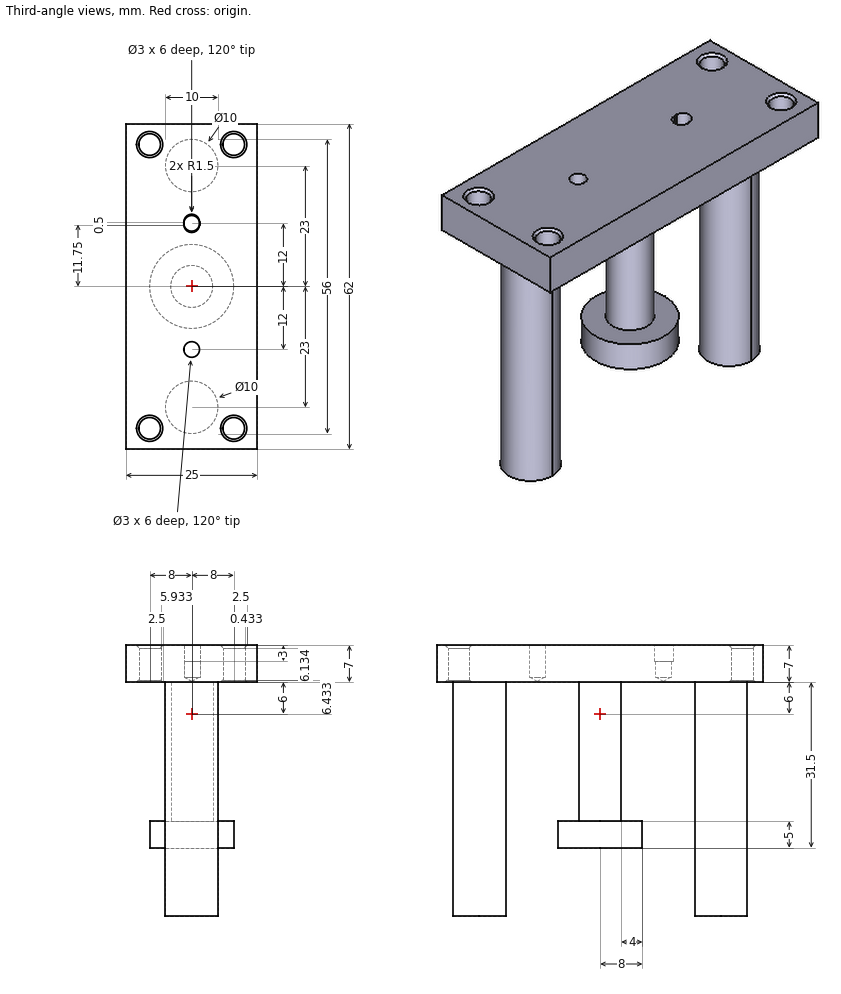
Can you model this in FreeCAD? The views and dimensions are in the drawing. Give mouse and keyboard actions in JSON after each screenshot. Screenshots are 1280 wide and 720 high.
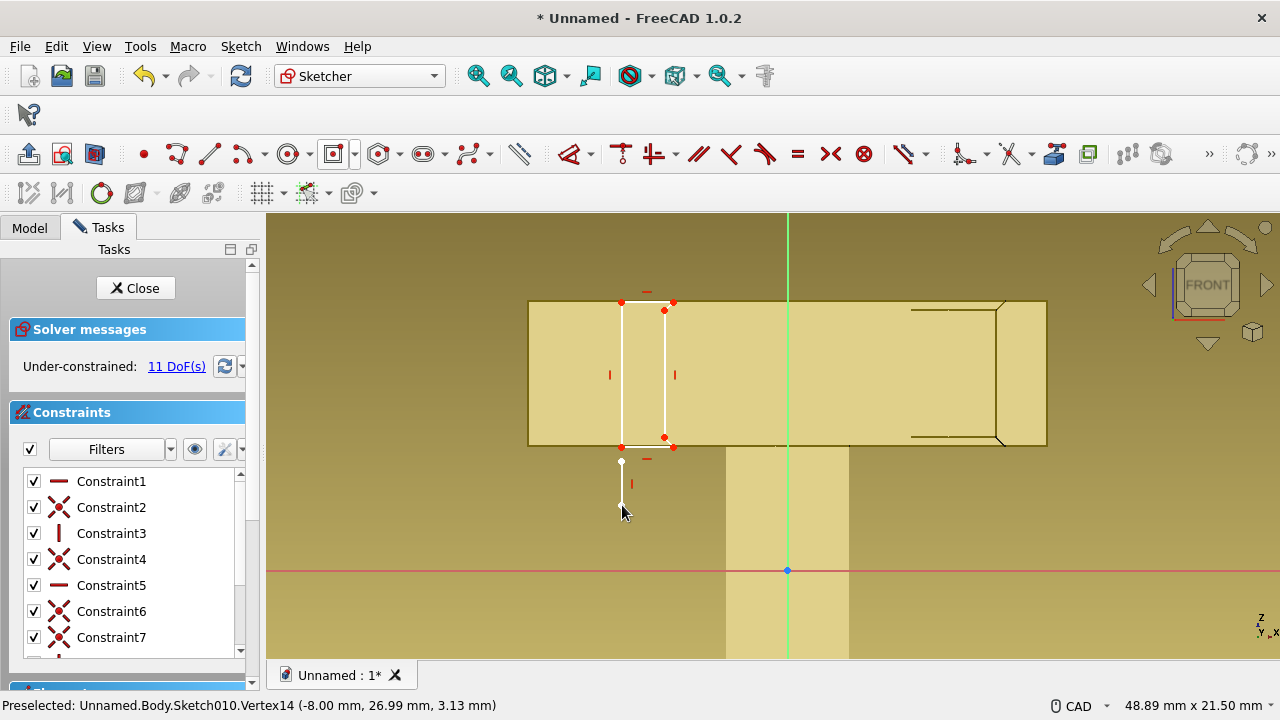
{"action": "left_click", "coordinate": [622, 475]}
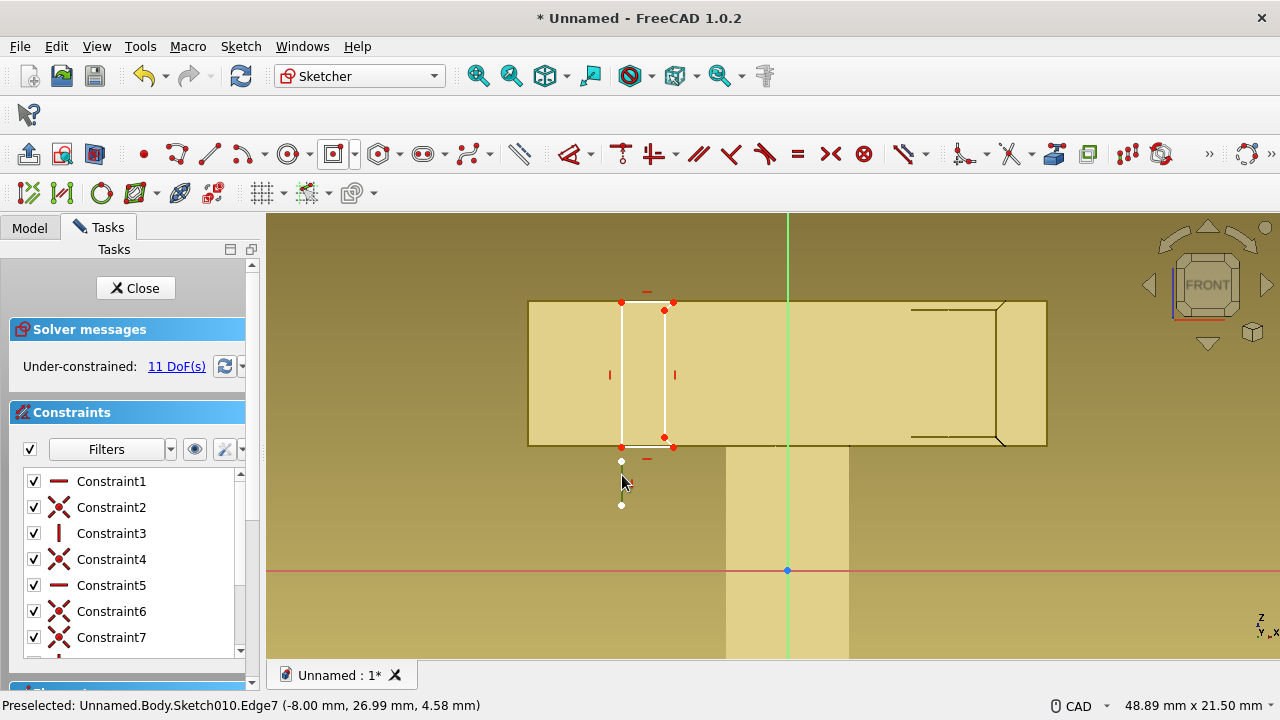
{"action": "left_click", "coordinate": [520, 154]}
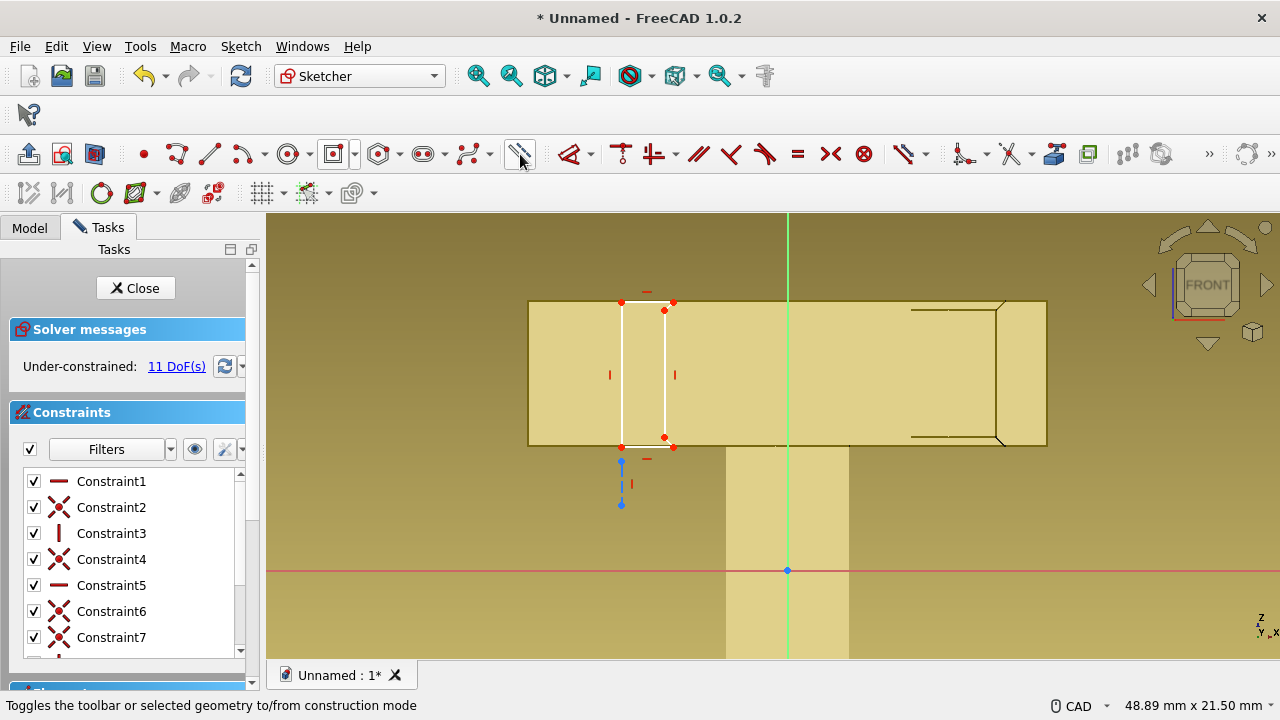
{"action": "left_click", "coordinate": [568, 154]}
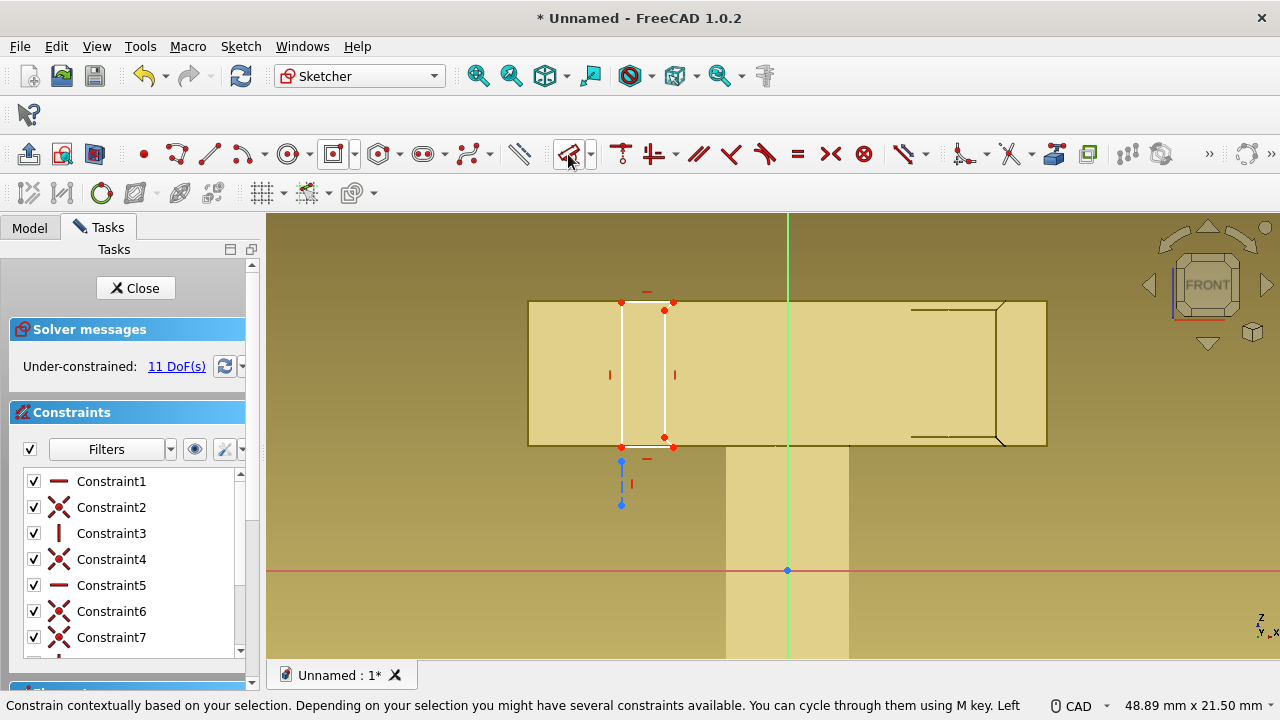
{"action": "left_click", "coordinate": [622, 404]}
{"action": "left_click", "coordinate": [588, 375]}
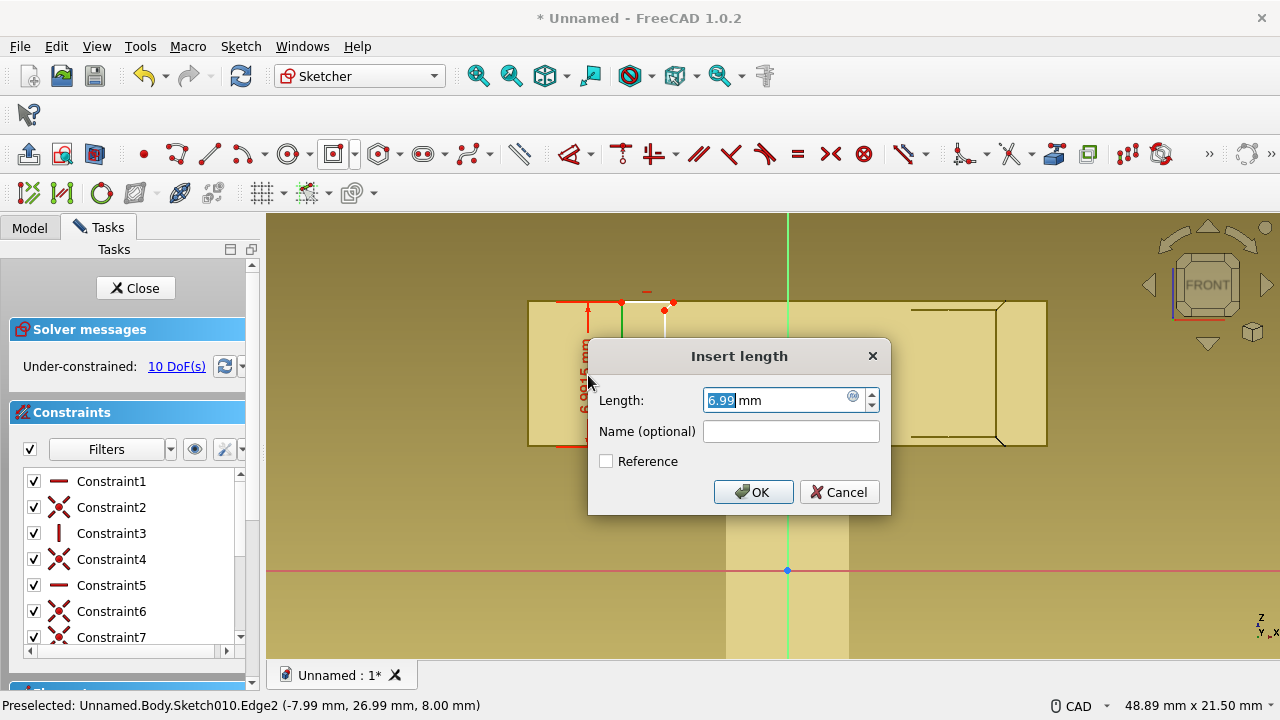
{"action": "type", "text": "7"}
{"action": "key", "text": "Return"}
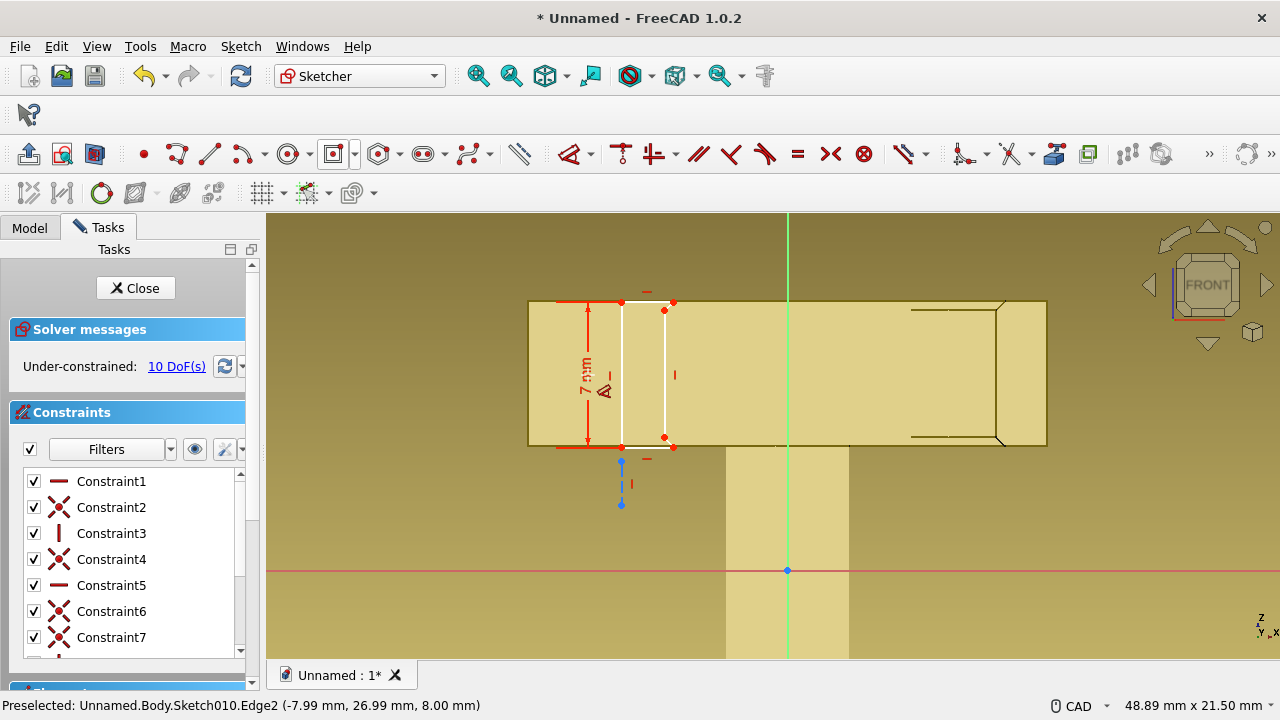
{"action": "left_click", "coordinate": [674, 448]}
{"action": "left_click", "coordinate": [822, 509]}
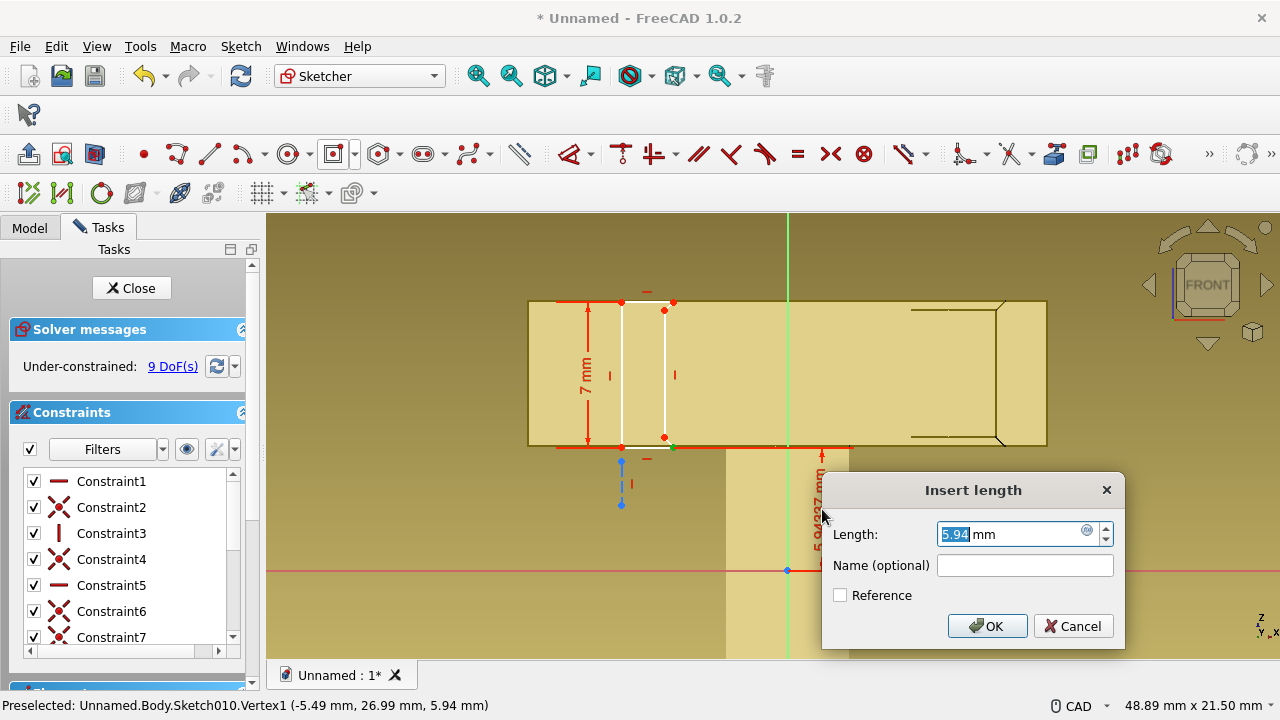
{"action": "type", "text": "6"}
{"action": "key", "text": "Return"}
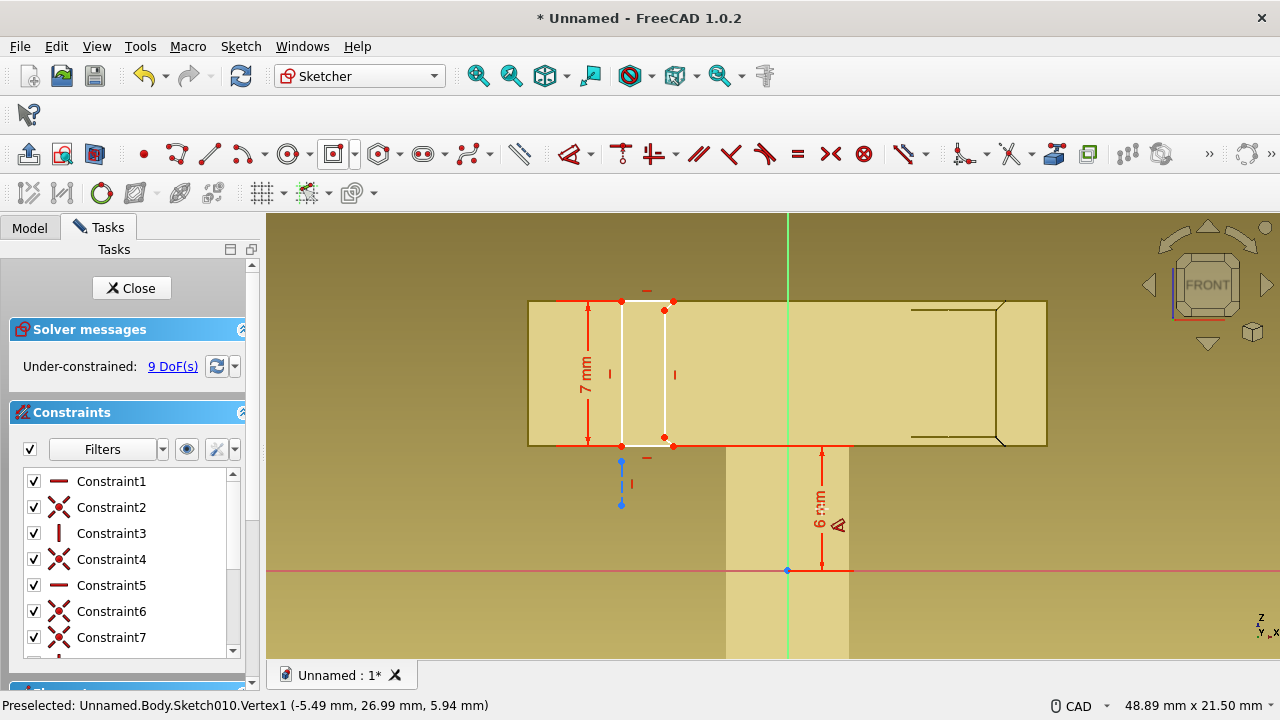
{"action": "left_click", "coordinate": [622, 446]}
{"action": "left_click", "coordinate": [705, 605]}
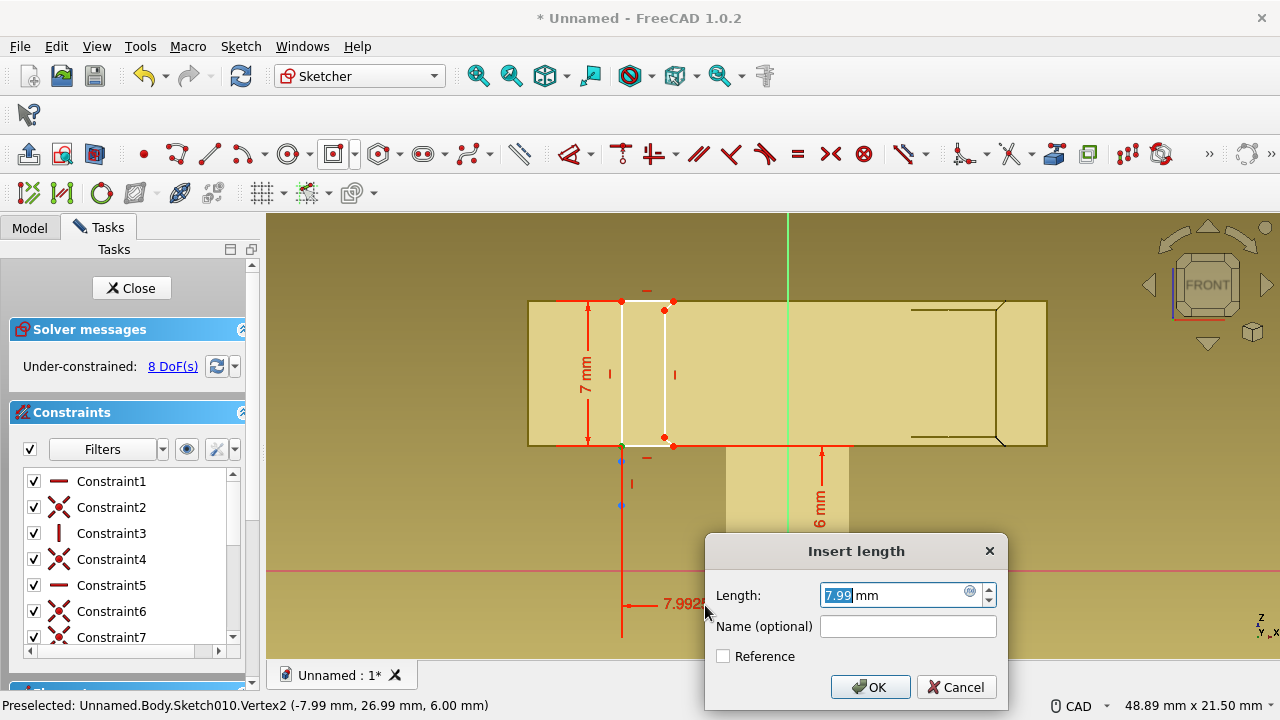
{"action": "type", "text": "8"}
{"action": "key", "text": "Return"}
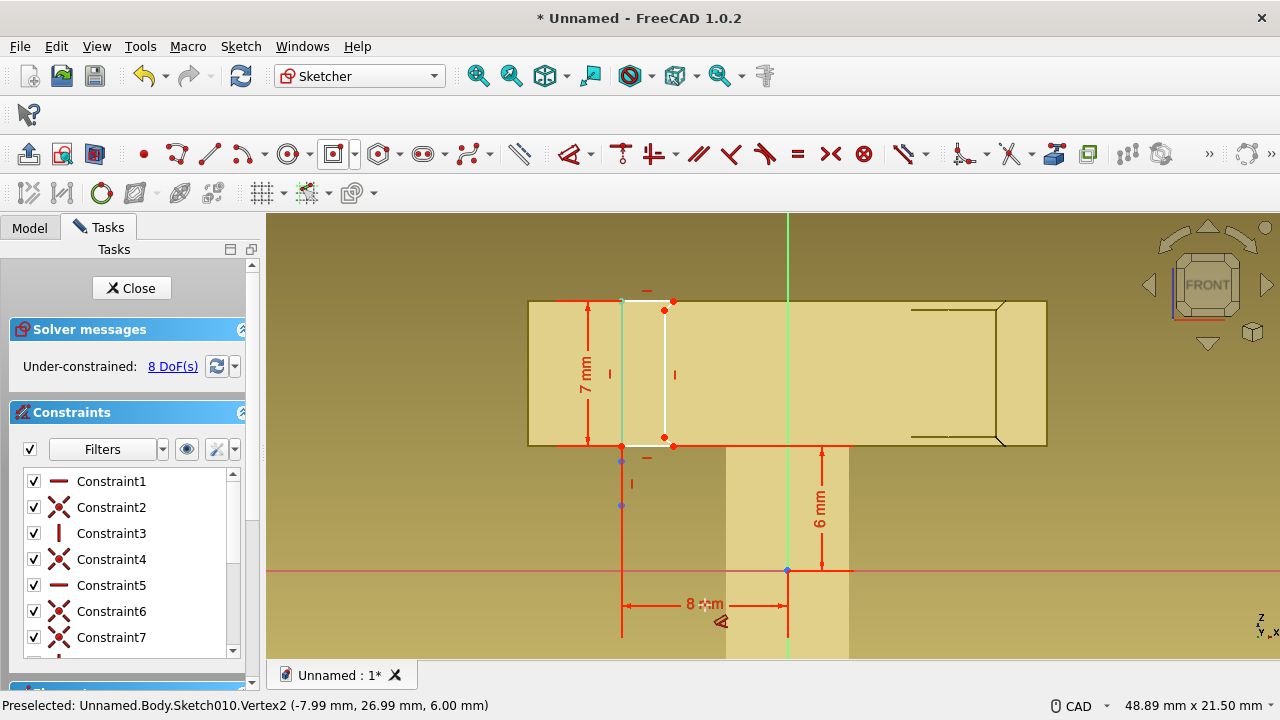
{"action": "left_click", "coordinate": [622, 461]}
{"action": "left_click", "coordinate": [705, 427]}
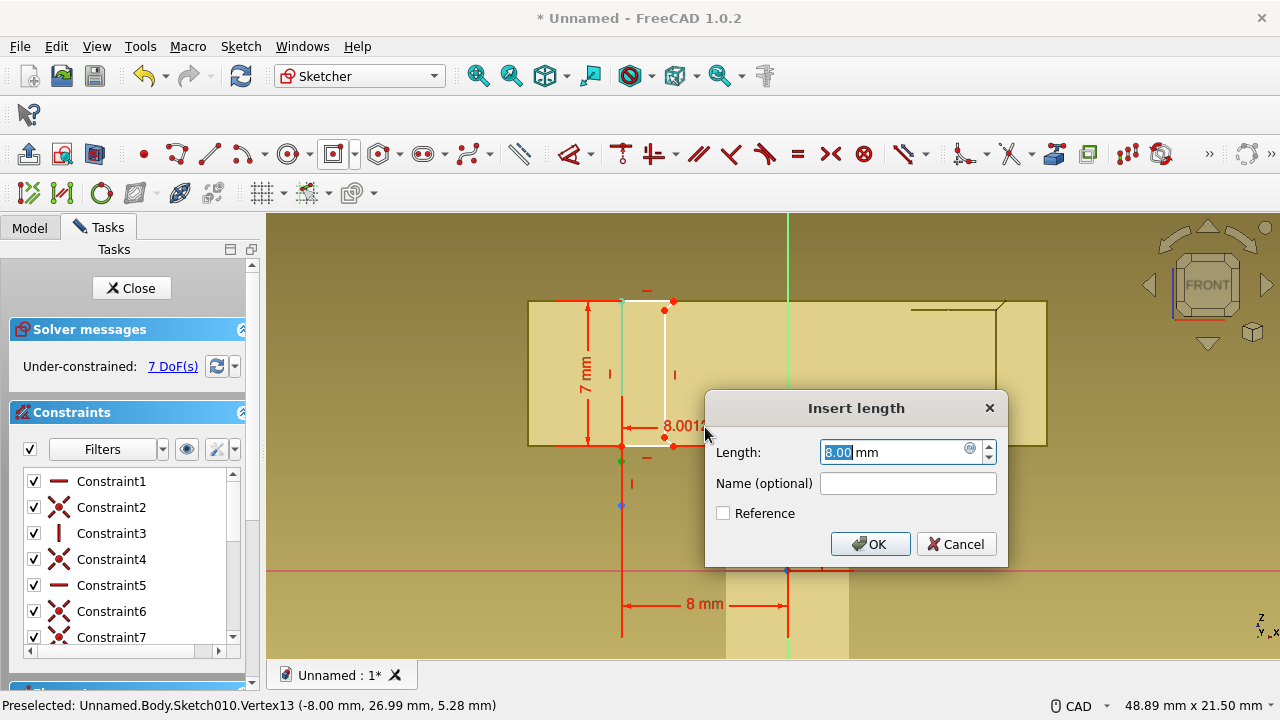
{"action": "type", "text": "8"}
{"action": "key", "text": "Return"}